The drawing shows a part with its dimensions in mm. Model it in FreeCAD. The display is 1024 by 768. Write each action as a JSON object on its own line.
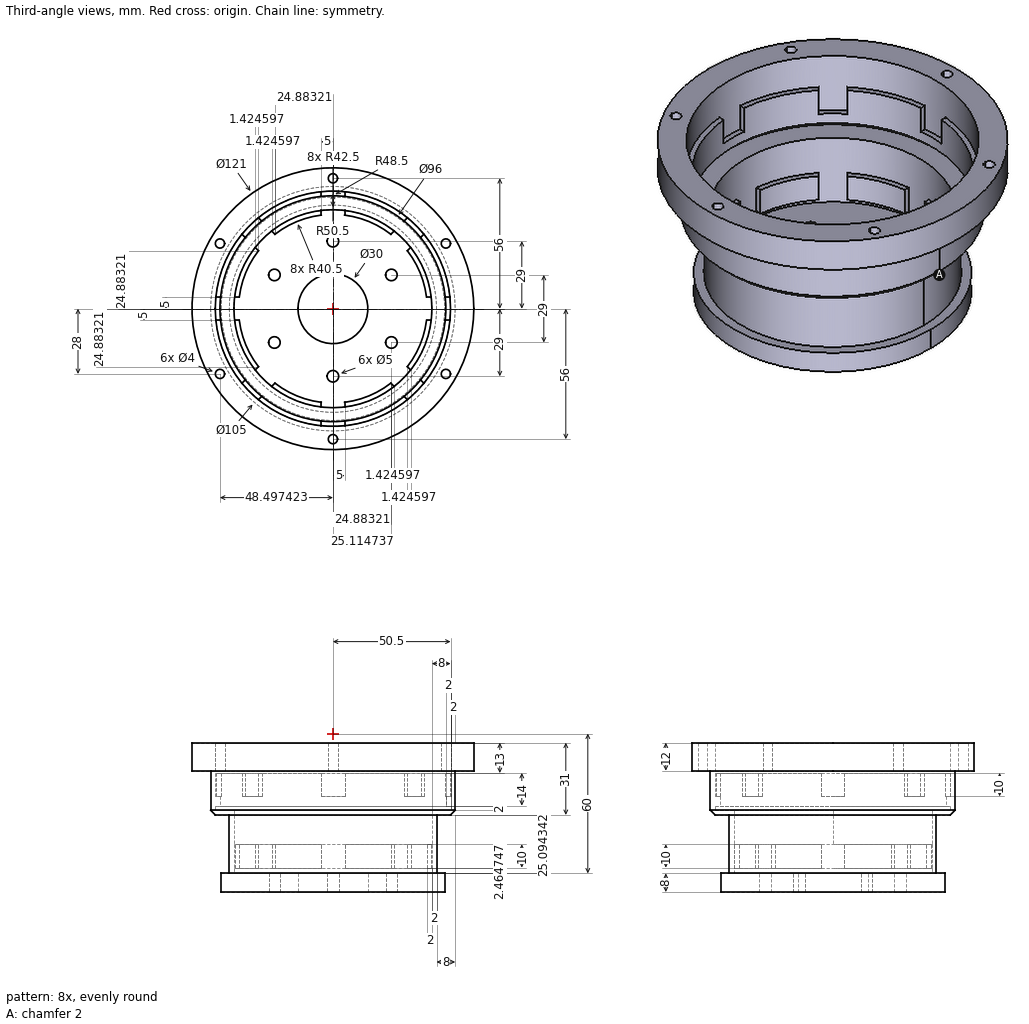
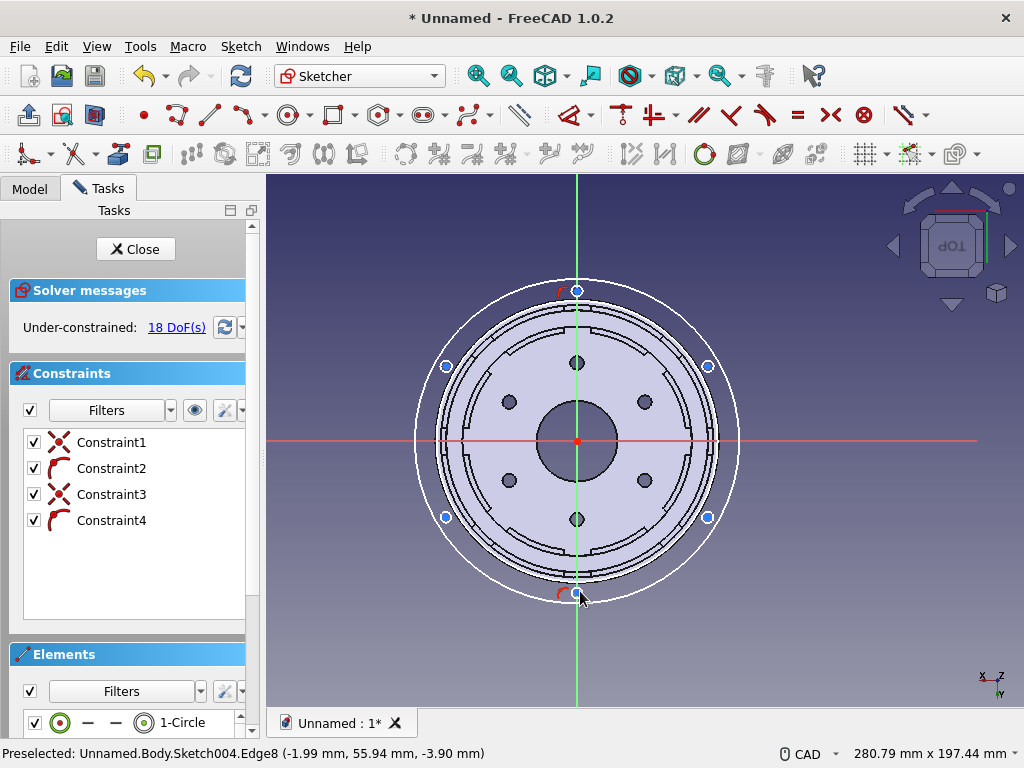
{"action": "scroll", "coordinate": [712, 362], "scroll_direction": "up", "scroll_amount": 5}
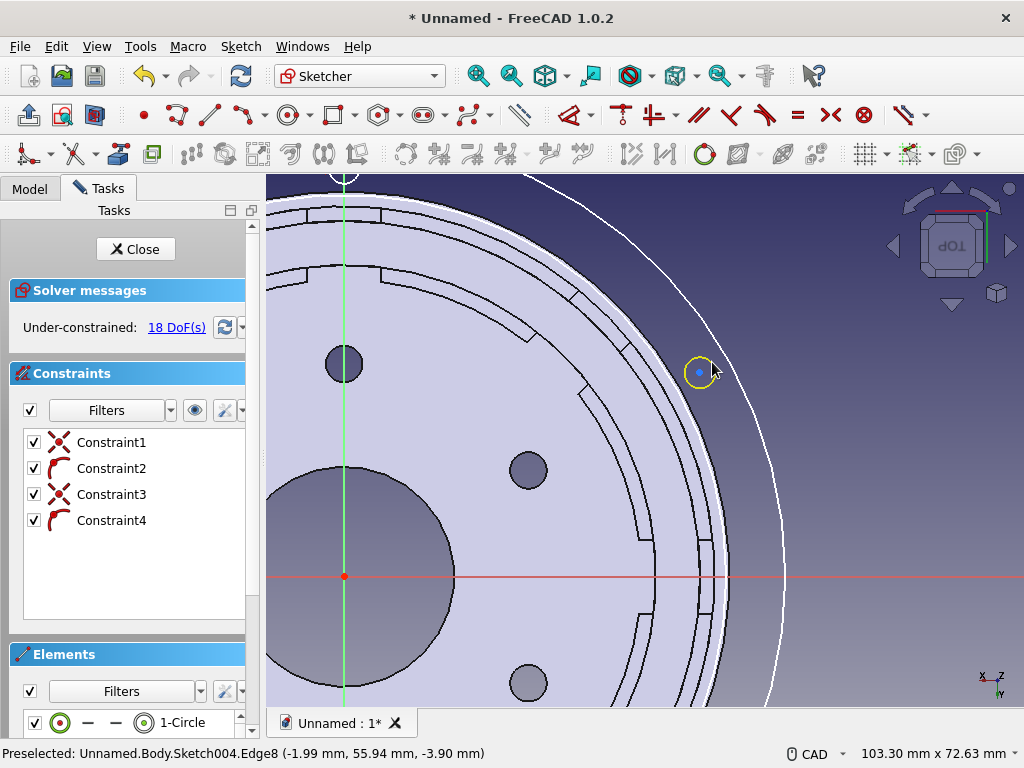
{"action": "left_click", "coordinate": [711, 362]}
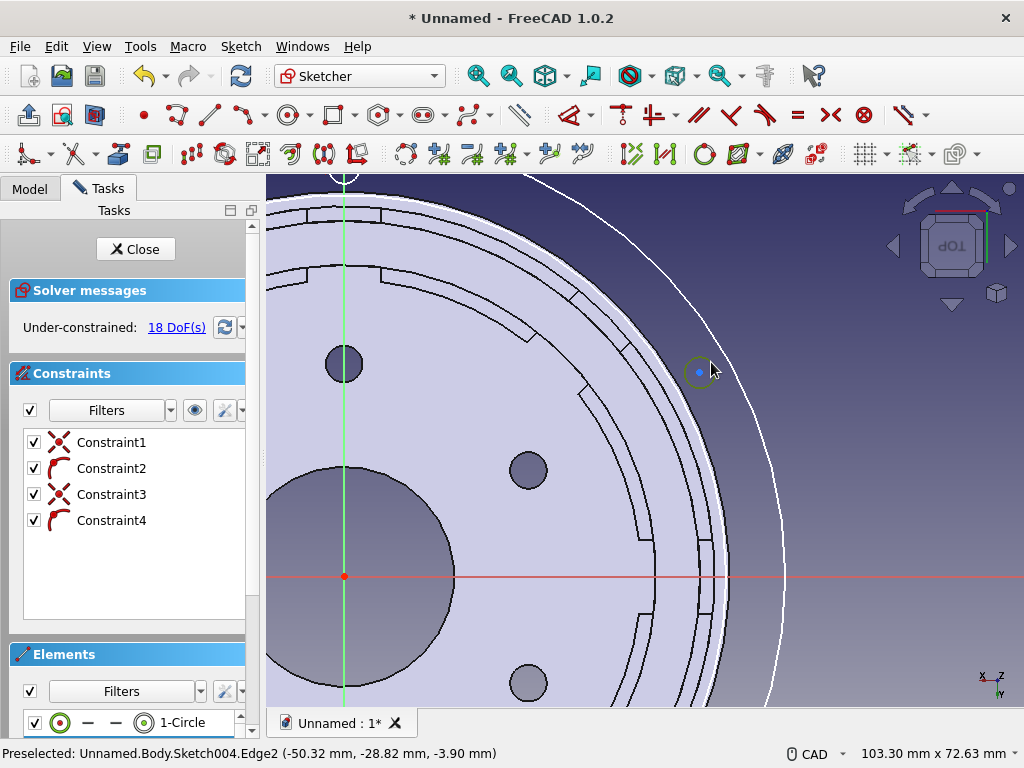
{"action": "scroll", "coordinate": [712, 361], "scroll_direction": "down", "scroll_amount": 5}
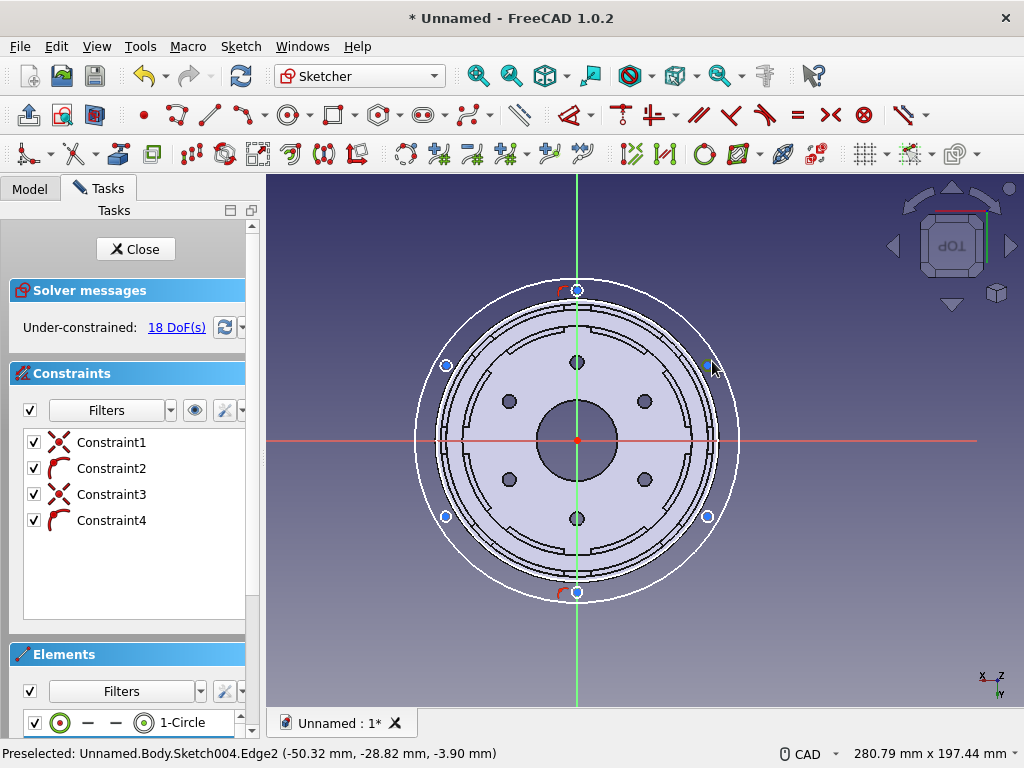
{"action": "scroll", "coordinate": [581, 286], "scroll_direction": "up", "scroll_amount": 7}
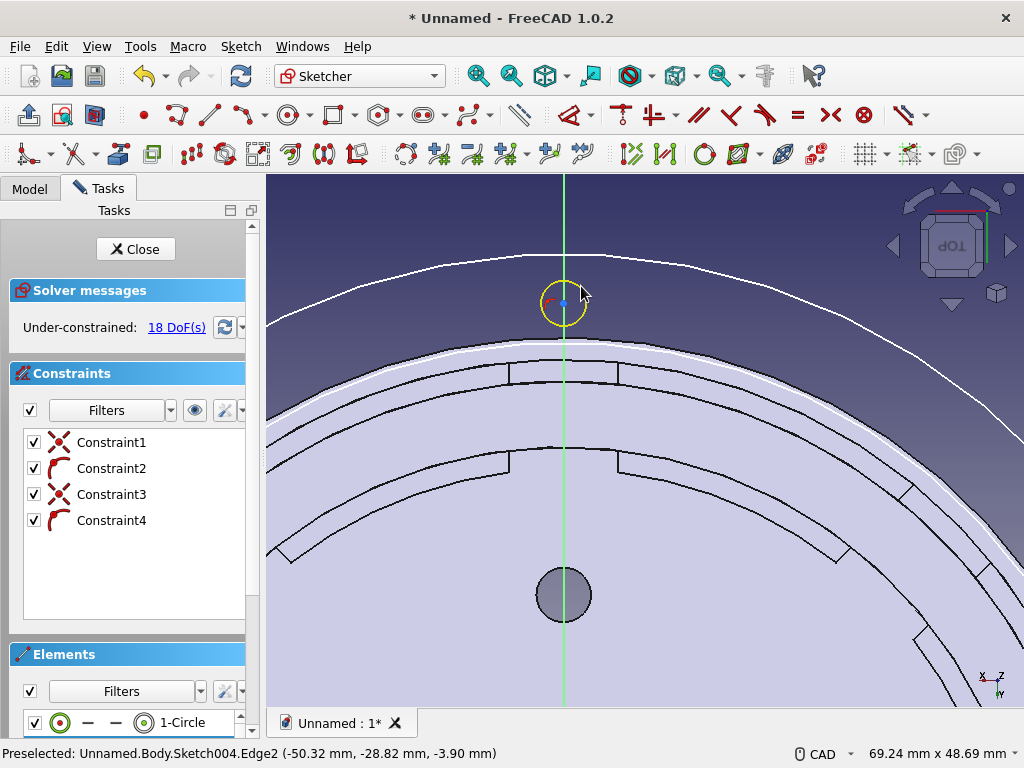
{"action": "left_click", "coordinate": [580, 287]}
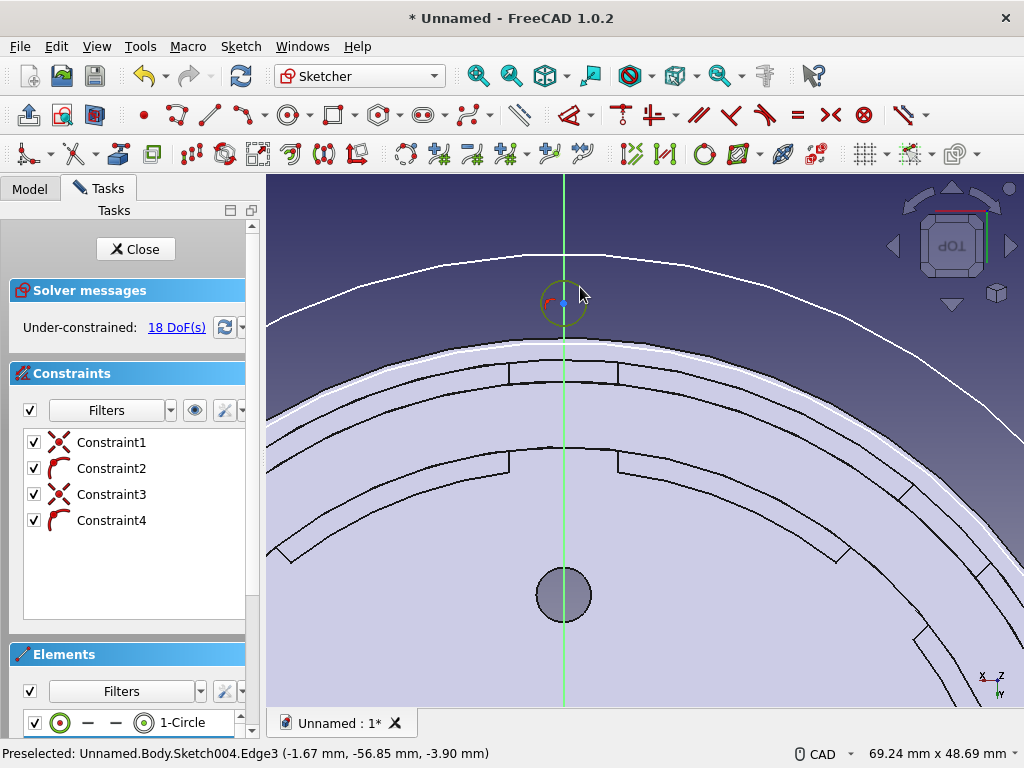
{"action": "scroll", "coordinate": [581, 286], "scroll_direction": "down", "scroll_amount": 7}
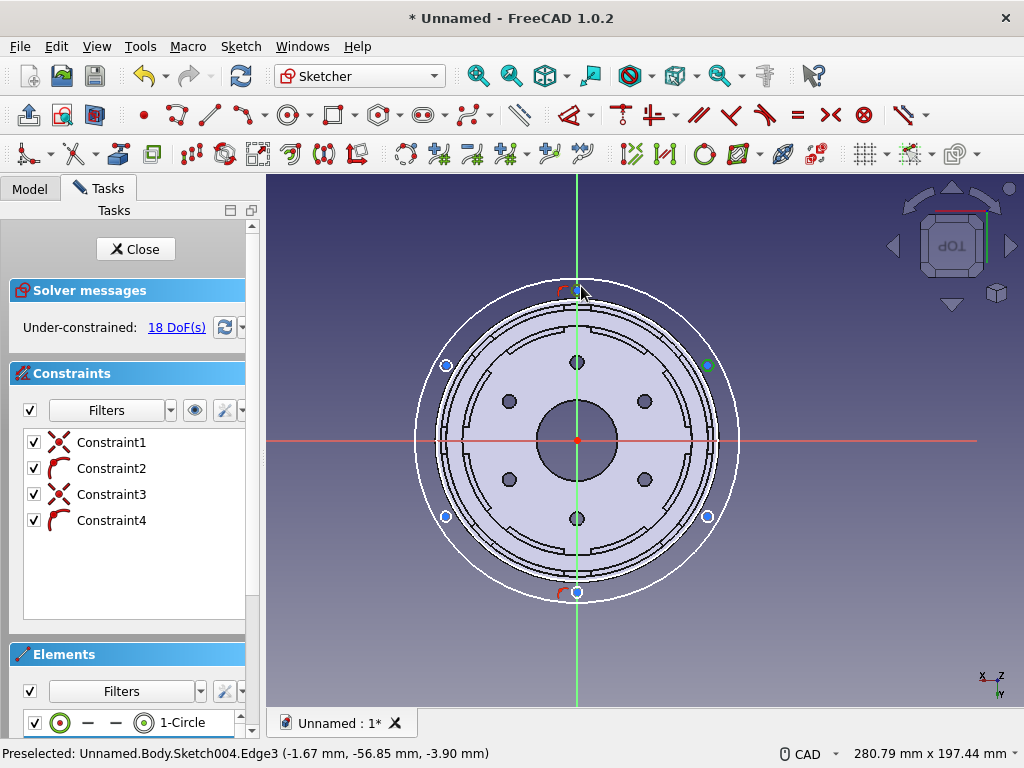
{"action": "scroll", "coordinate": [450, 362], "scroll_direction": "up", "scroll_amount": 5}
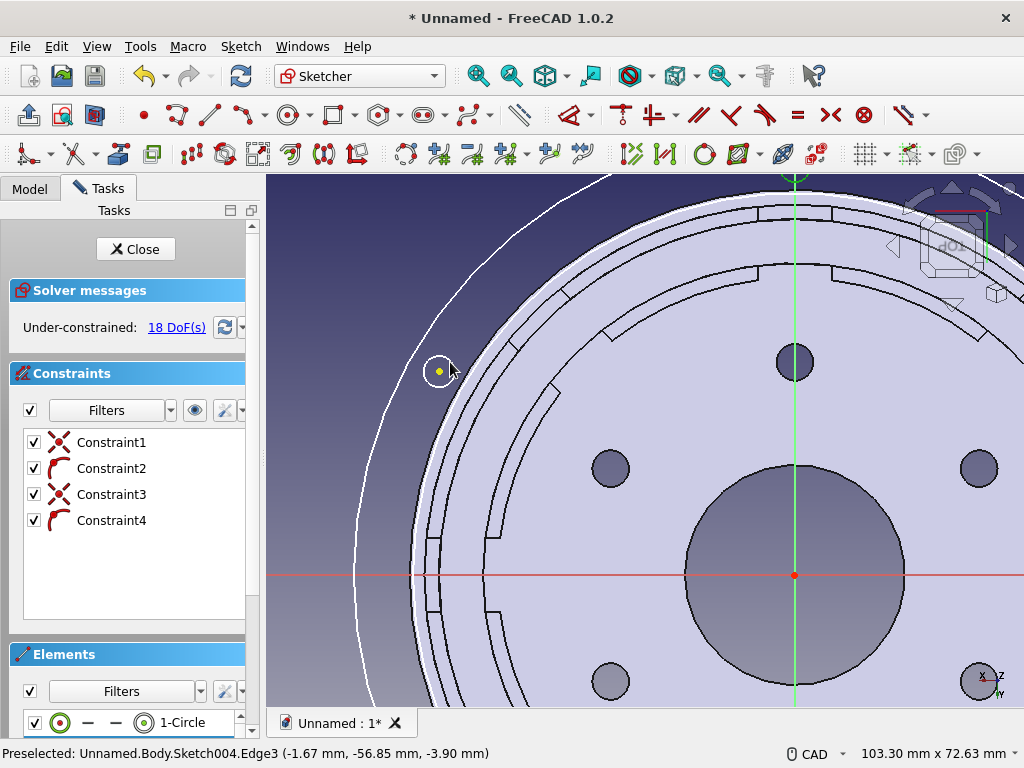
{"action": "left_click", "coordinate": [450, 361]}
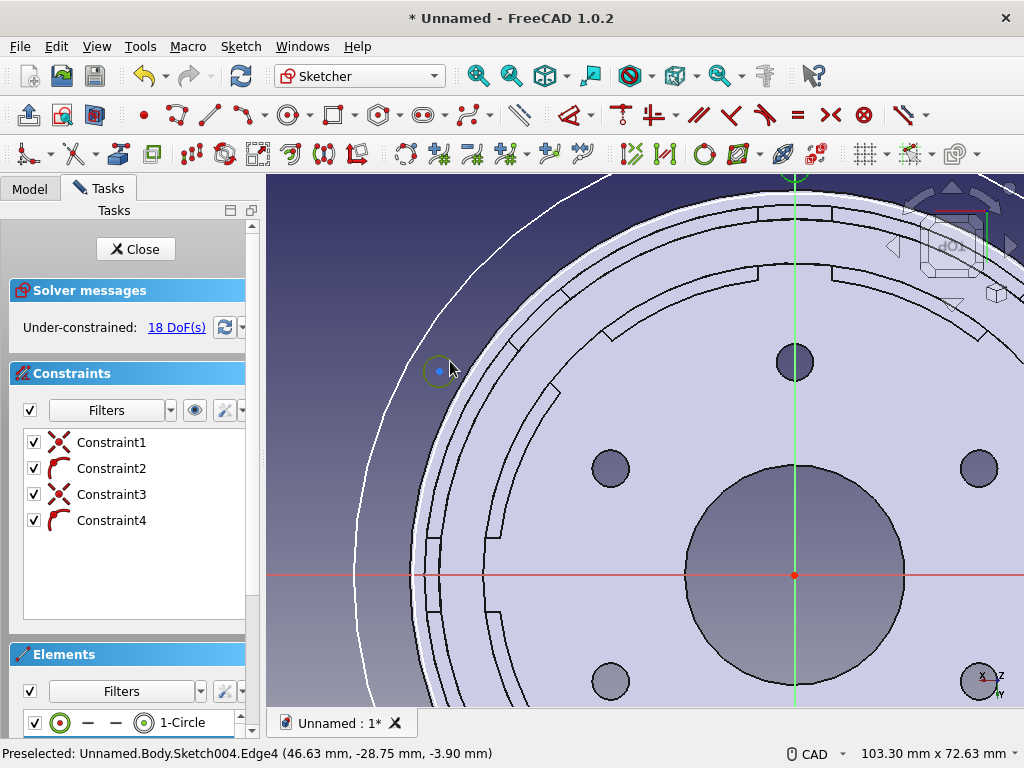
{"action": "scroll", "coordinate": [449, 362], "scroll_direction": "down", "scroll_amount": 5}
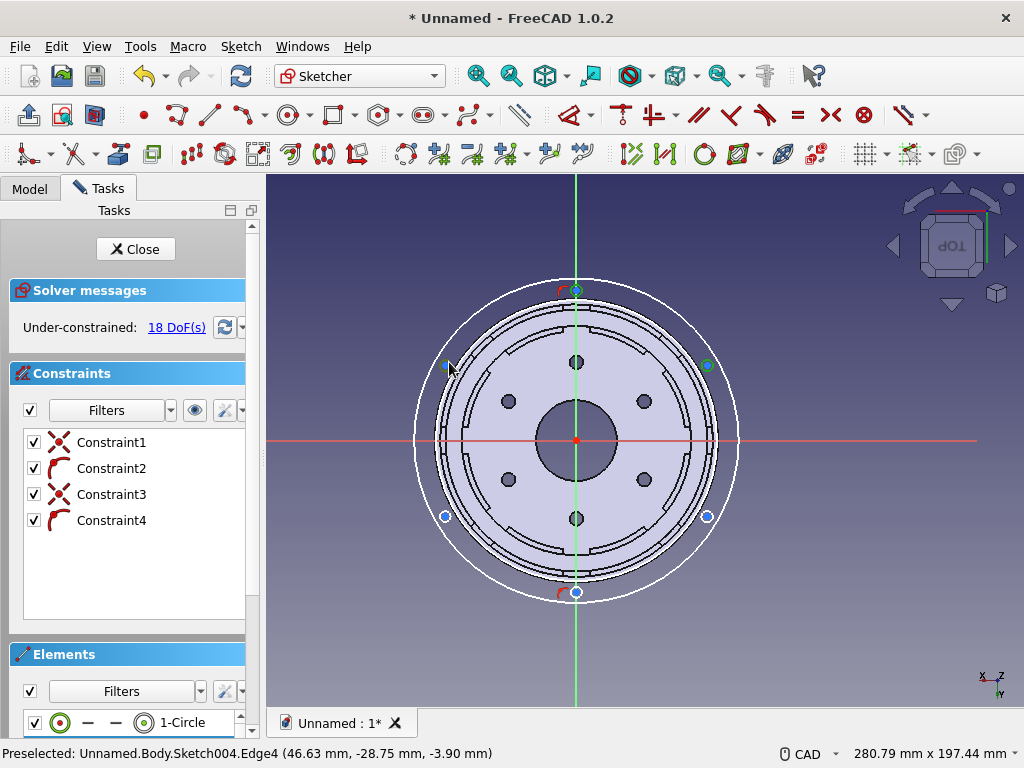
{"action": "scroll", "coordinate": [711, 513], "scroll_direction": "up", "scroll_amount": 5}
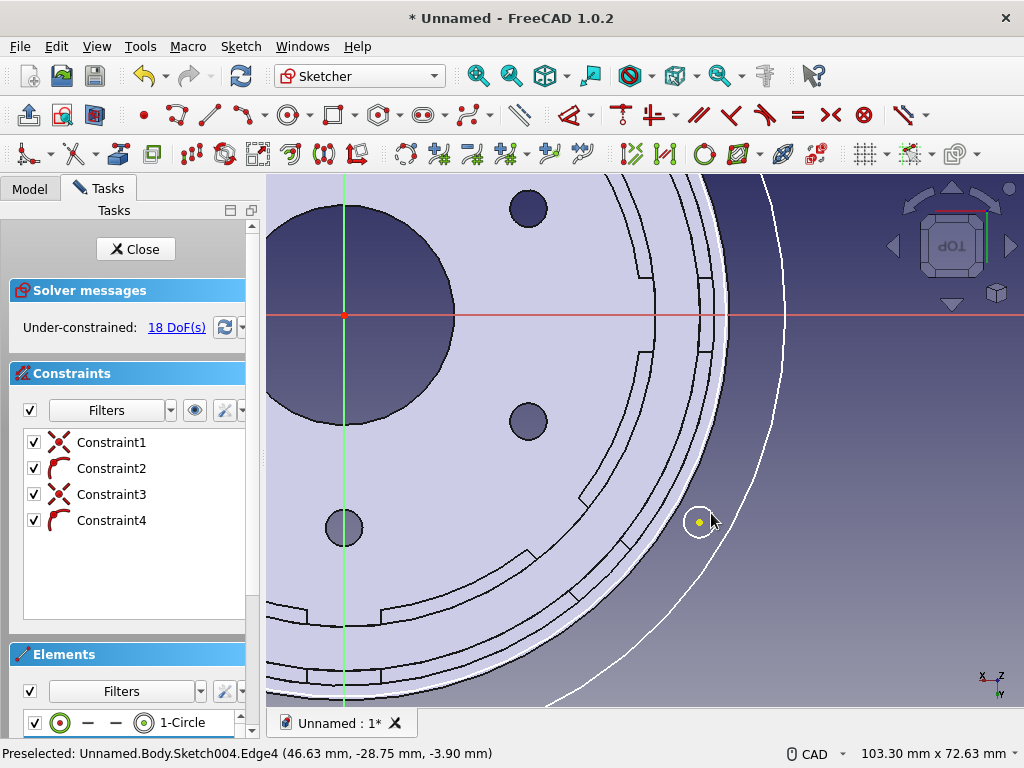
{"action": "left_click", "coordinate": [710, 511]}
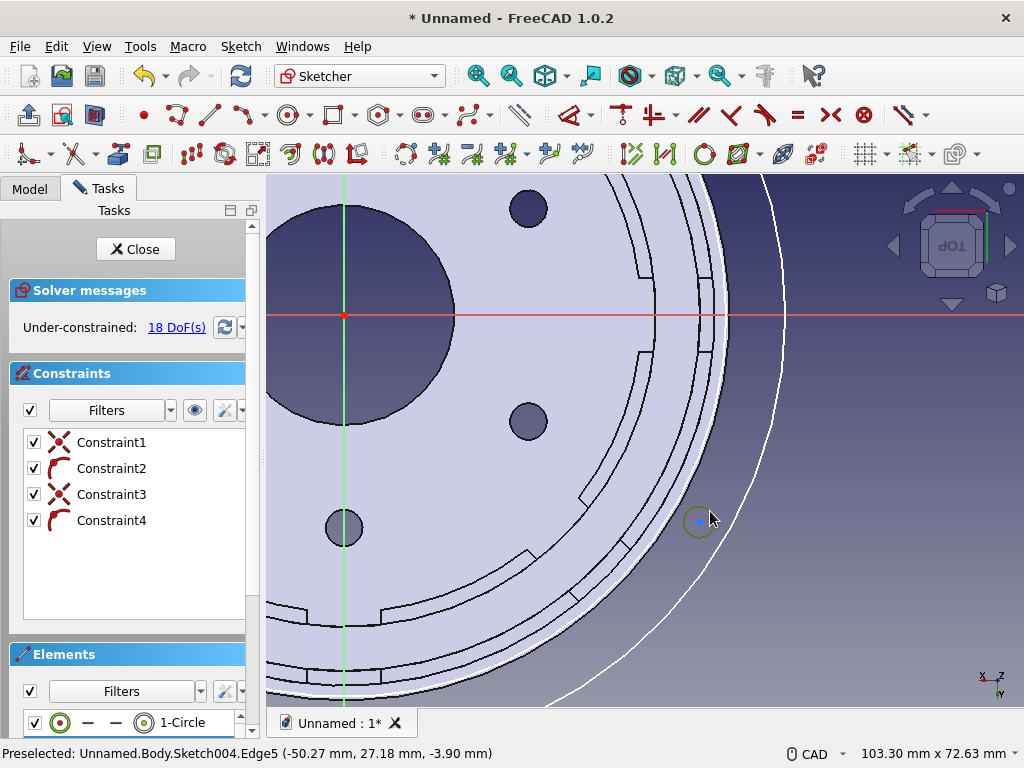
{"action": "scroll", "coordinate": [712, 513], "scroll_direction": "down", "scroll_amount": 5}